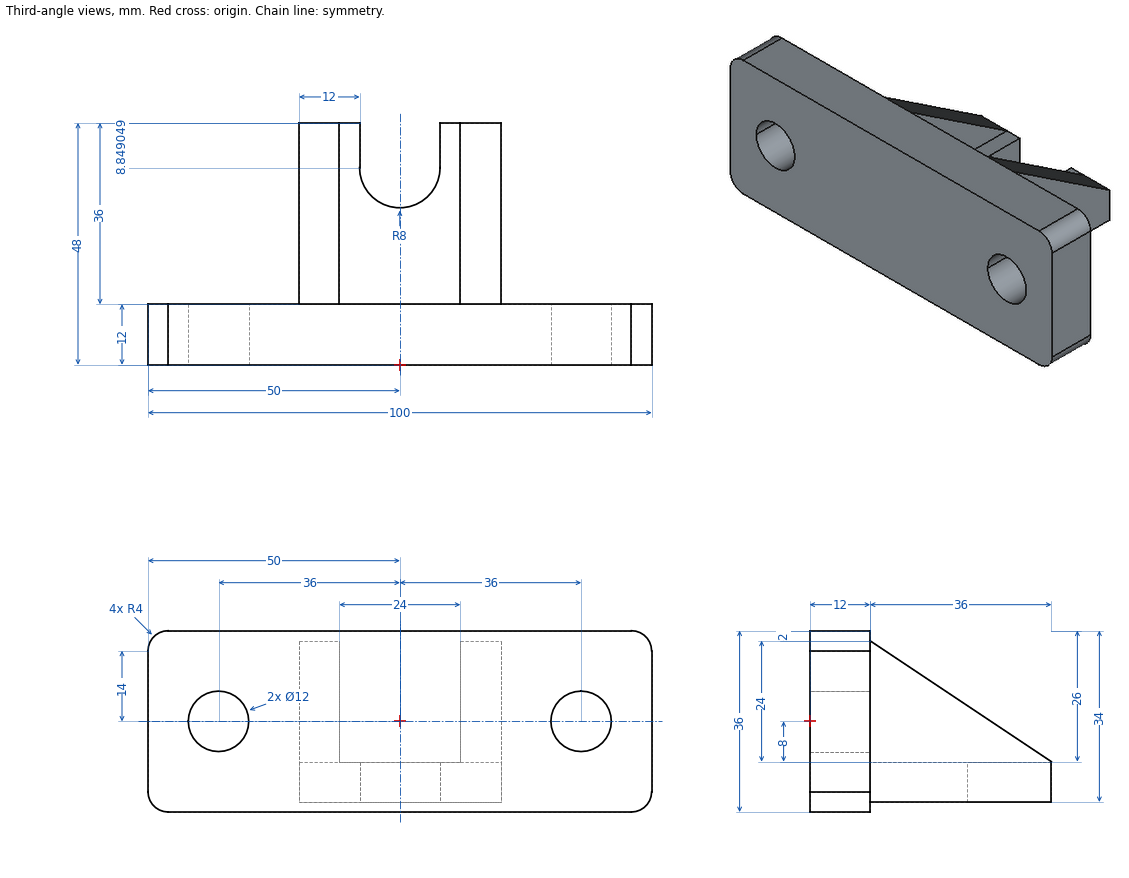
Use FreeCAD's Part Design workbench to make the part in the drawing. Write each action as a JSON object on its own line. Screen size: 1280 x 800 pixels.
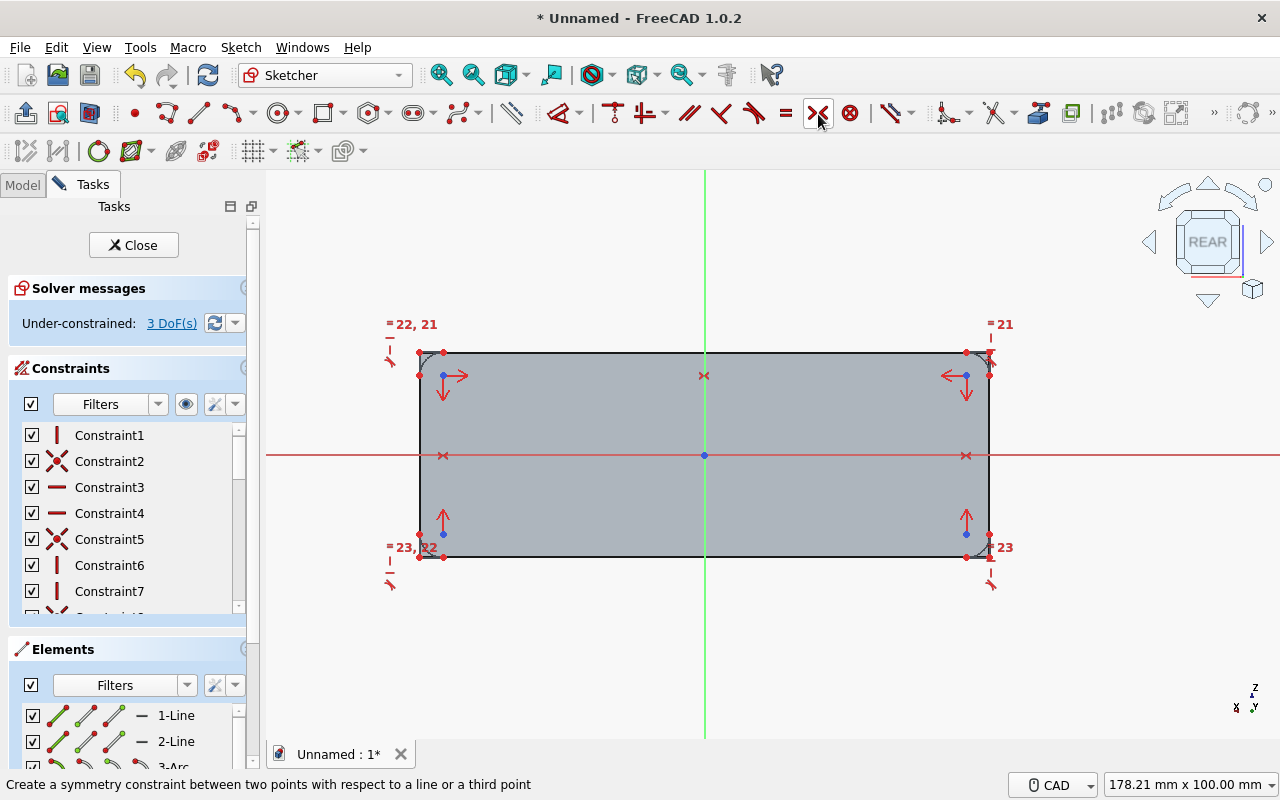
{"action": "left_click", "coordinate": [558, 114]}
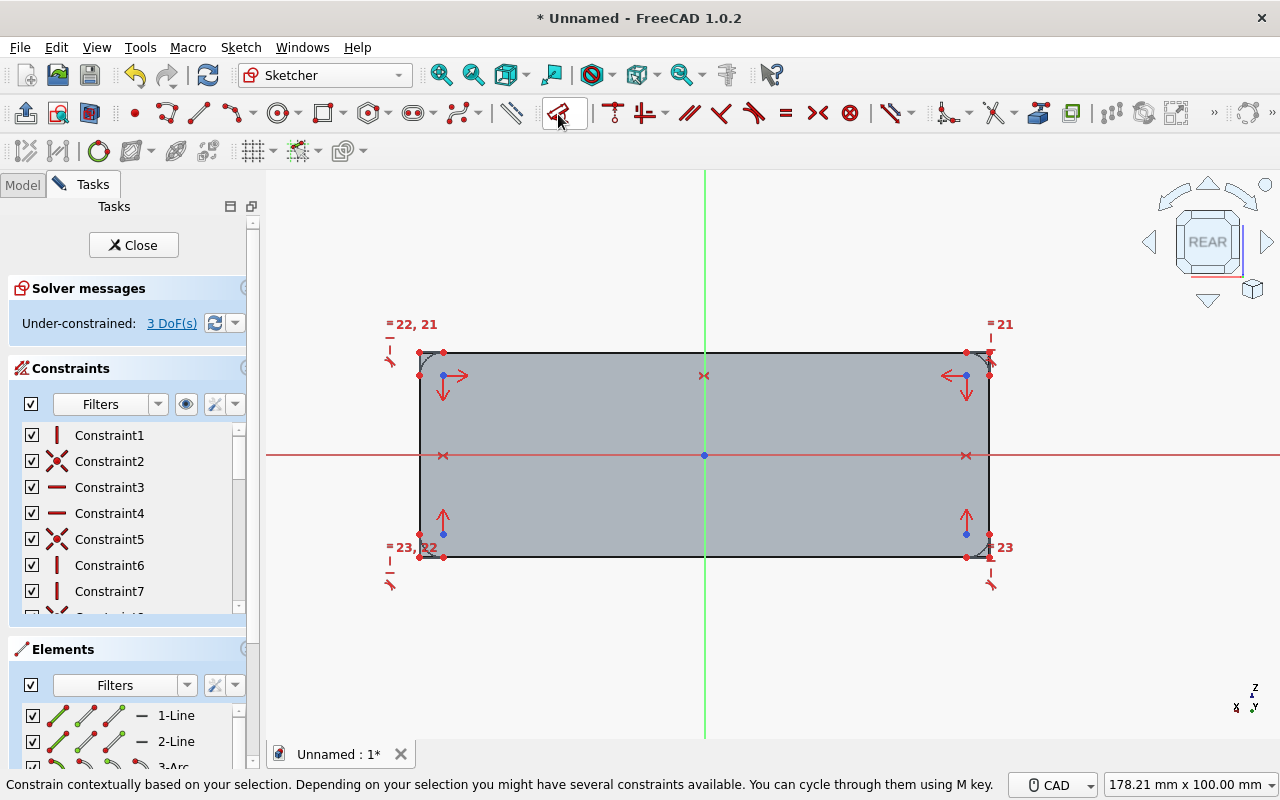
{"action": "scroll", "coordinate": [983, 359], "scroll_direction": "up", "scroll_amount": 4}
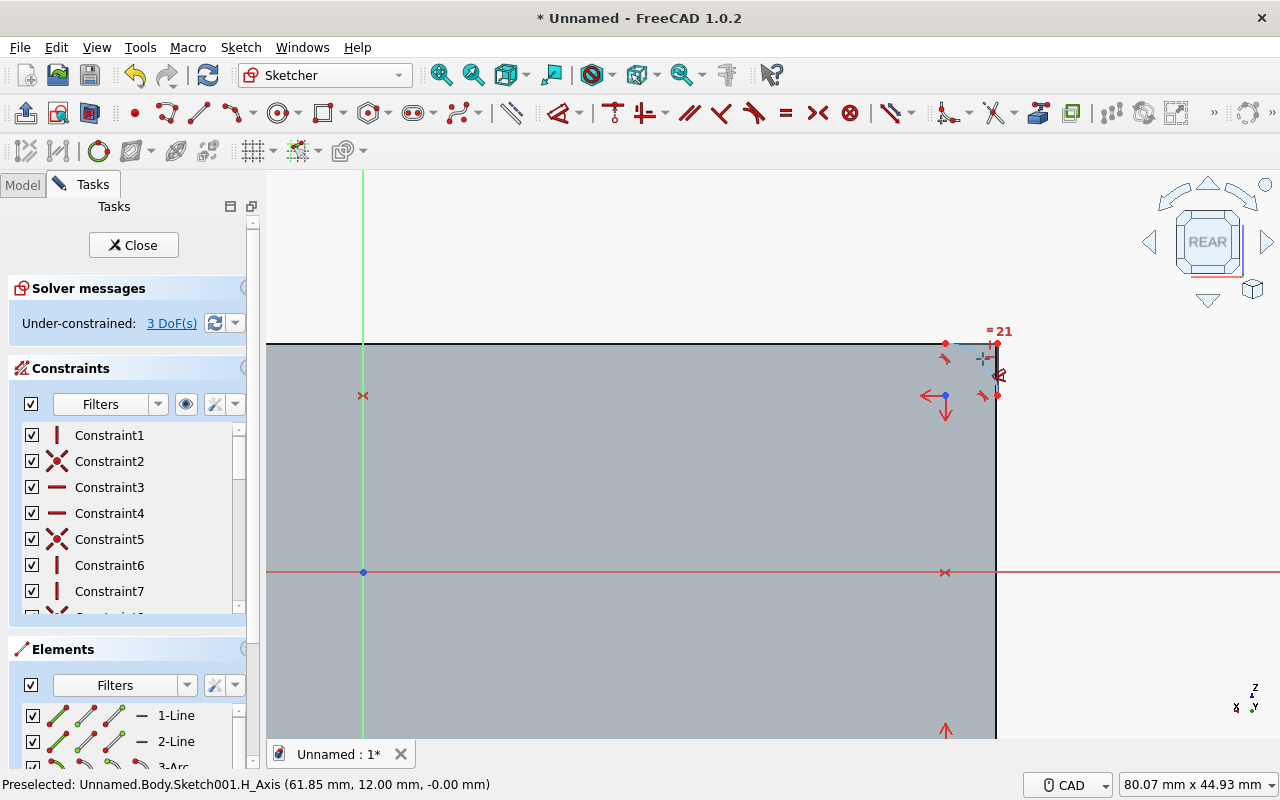
{"action": "left_click", "coordinate": [982, 359]}
{"action": "left_click", "coordinate": [1026, 372]}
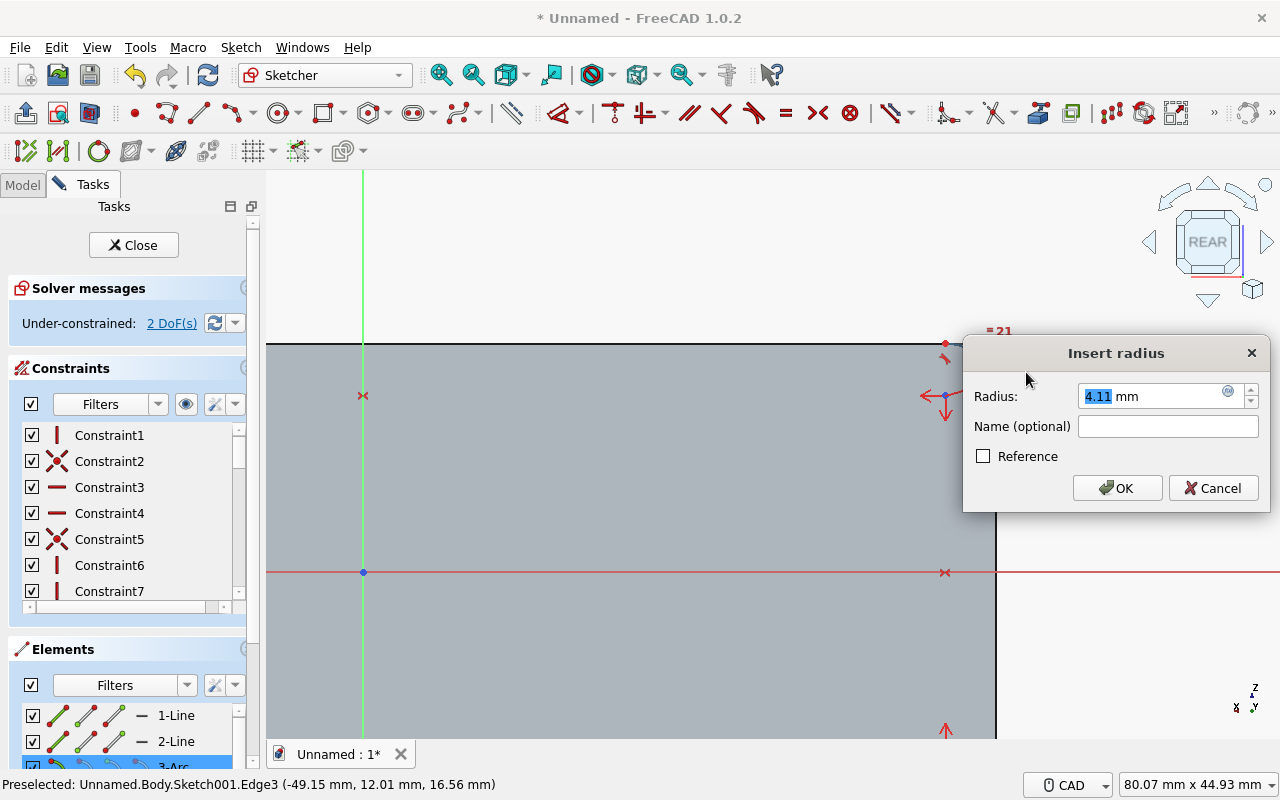
{"action": "type", "text": "4"}
{"action": "key", "text": "Return"}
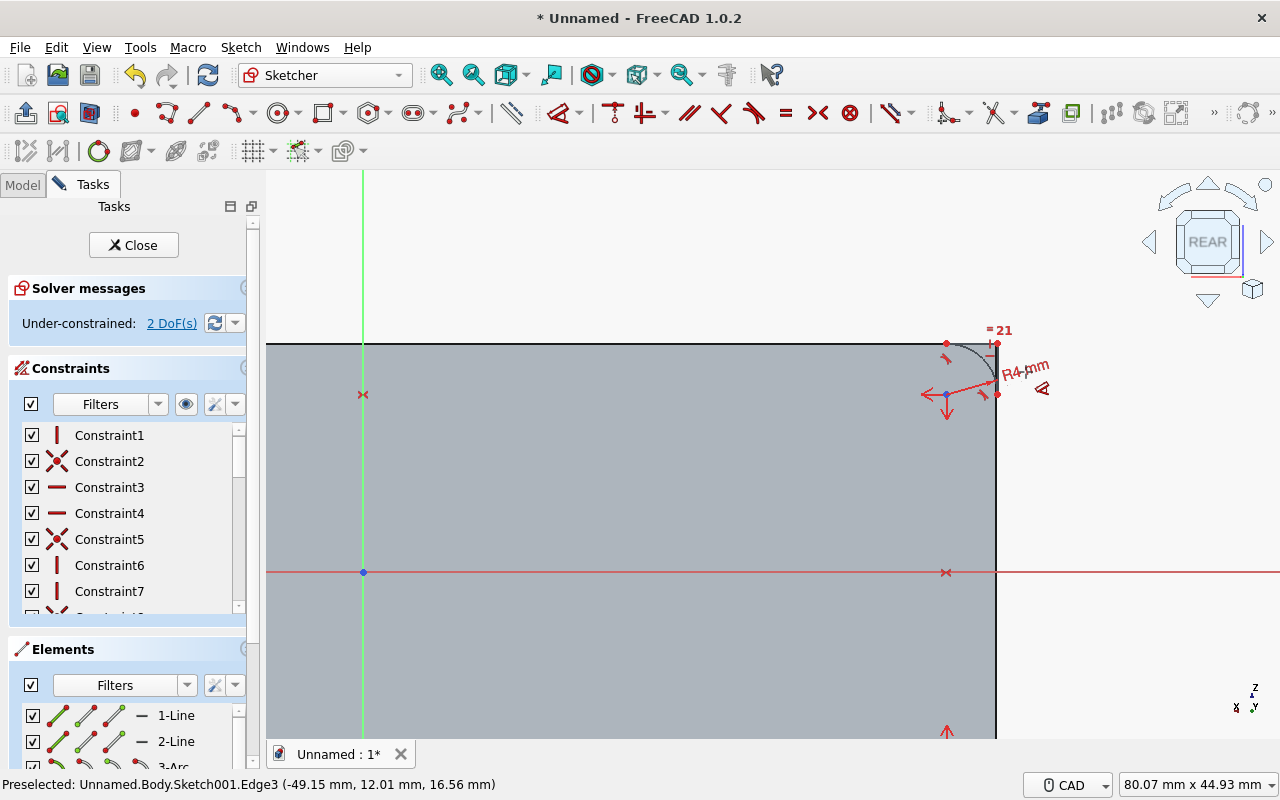
{"action": "left_click", "coordinate": [998, 395]}
{"action": "left_click", "coordinate": [680, 361]}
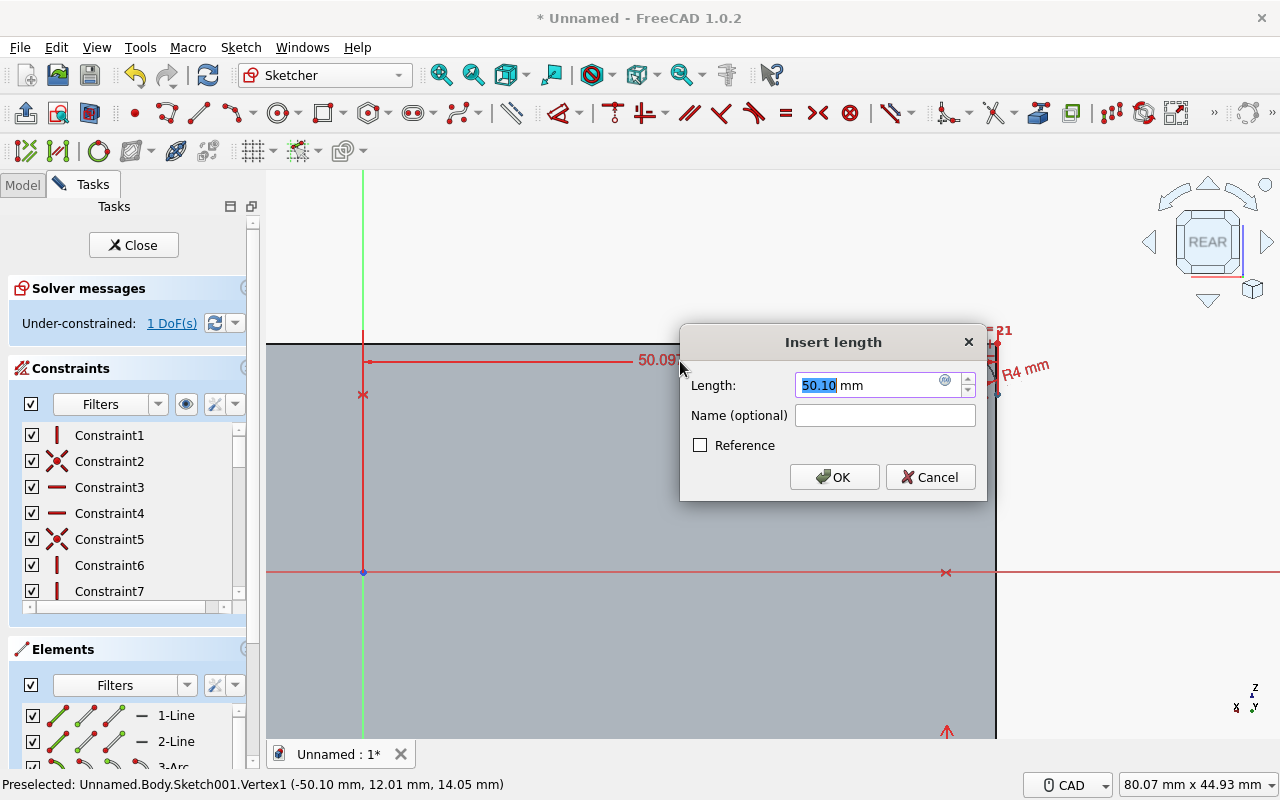
{"action": "type", "text": "50"}
{"action": "key", "text": "Return"}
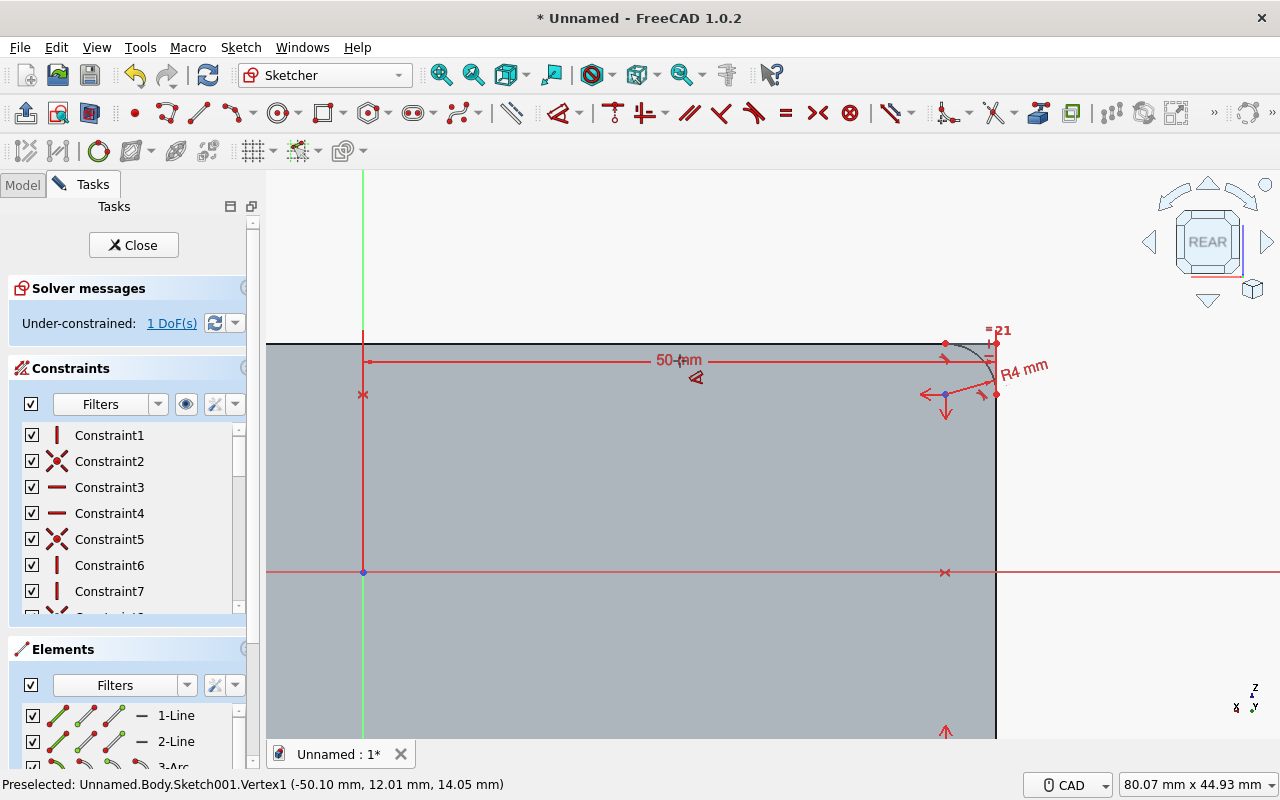
{"action": "left_click", "coordinate": [996, 395]}
{"action": "left_click", "coordinate": [1030, 483]}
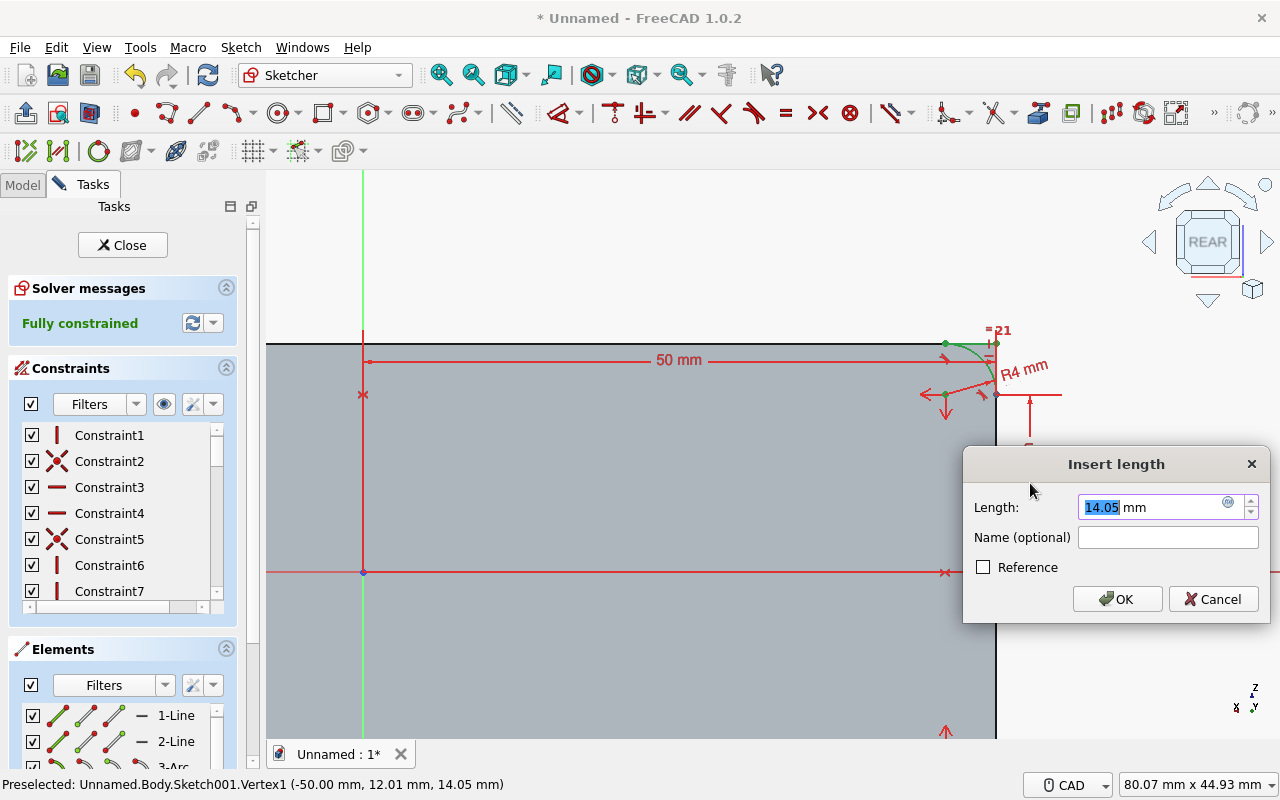
{"action": "type", "text": "14"}
{"action": "key", "text": "Return"}
{"action": "key", "text": "Escape"}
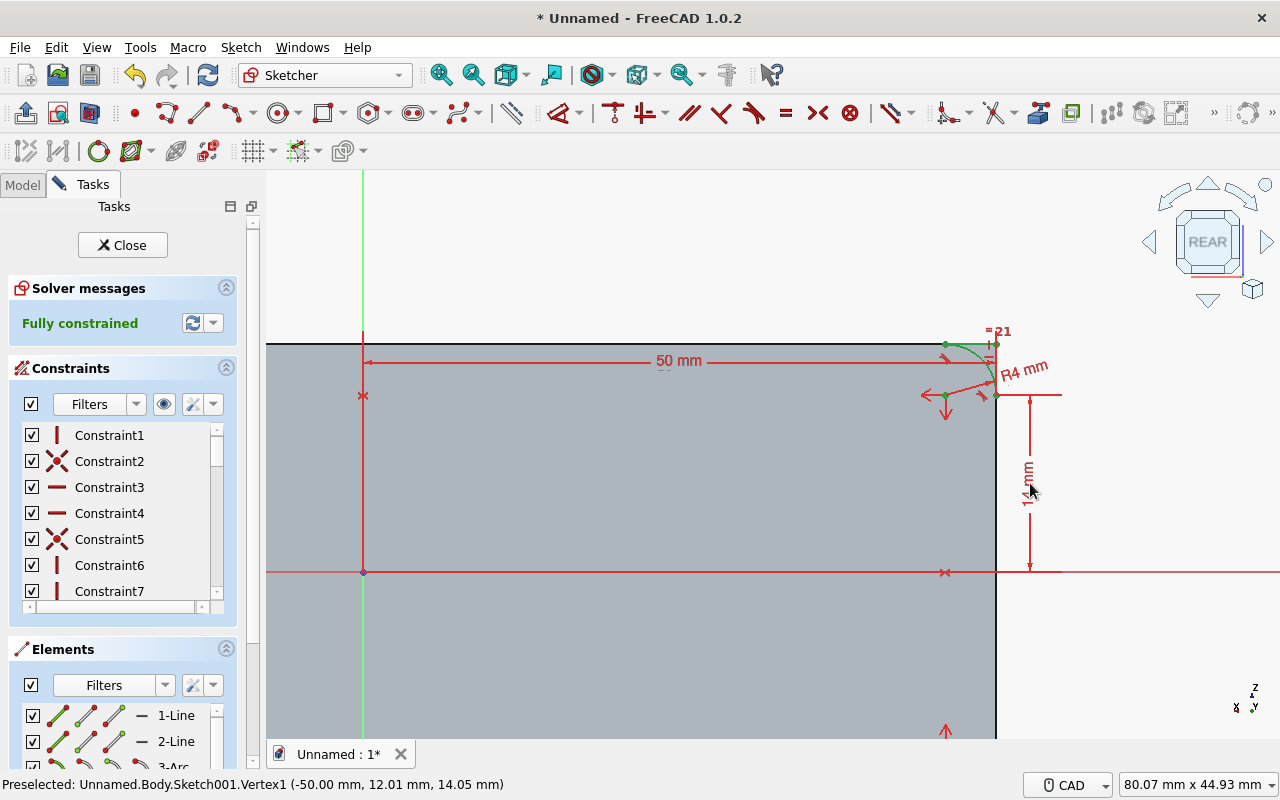
{"action": "left_click", "coordinate": [123, 245]}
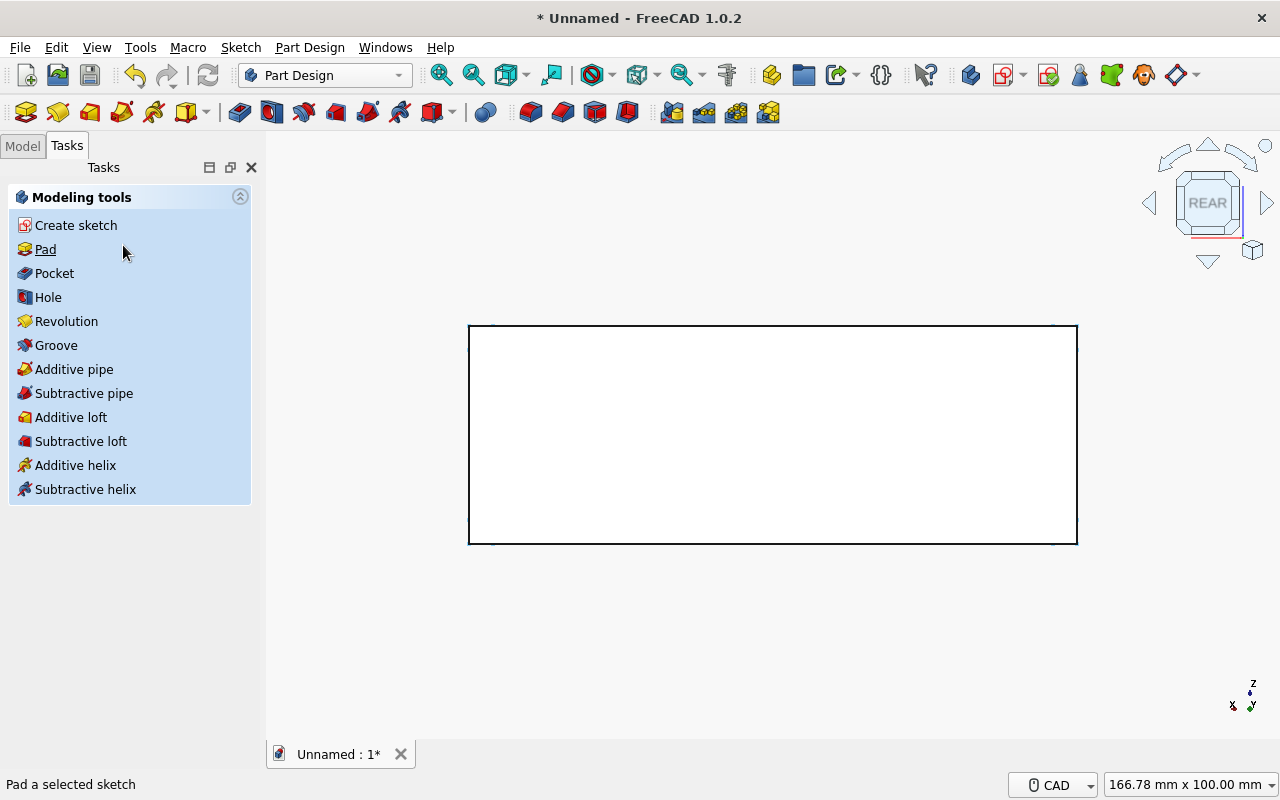
{"action": "left_click", "coordinate": [240, 112]}